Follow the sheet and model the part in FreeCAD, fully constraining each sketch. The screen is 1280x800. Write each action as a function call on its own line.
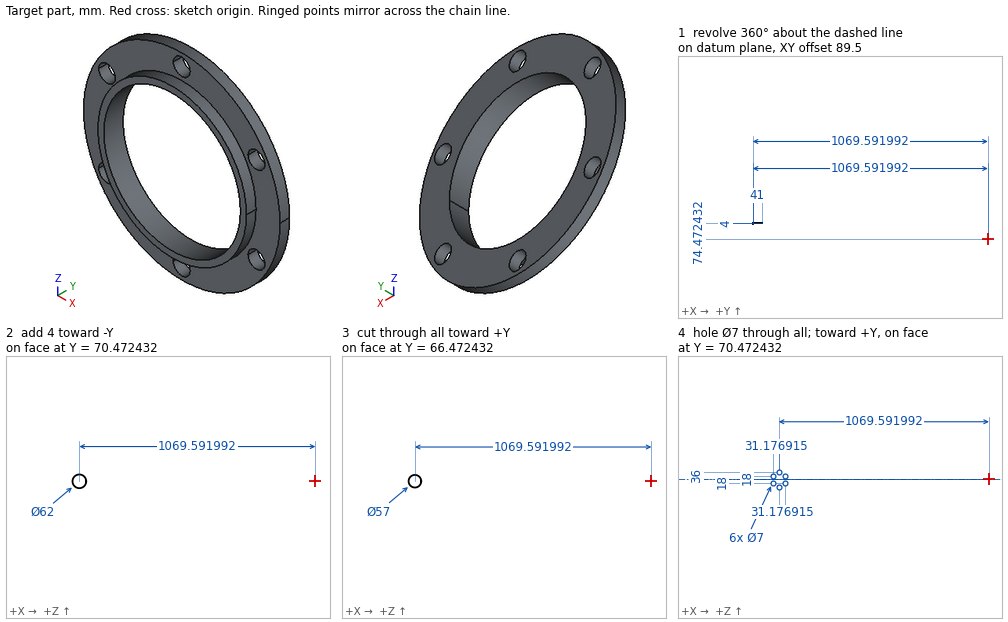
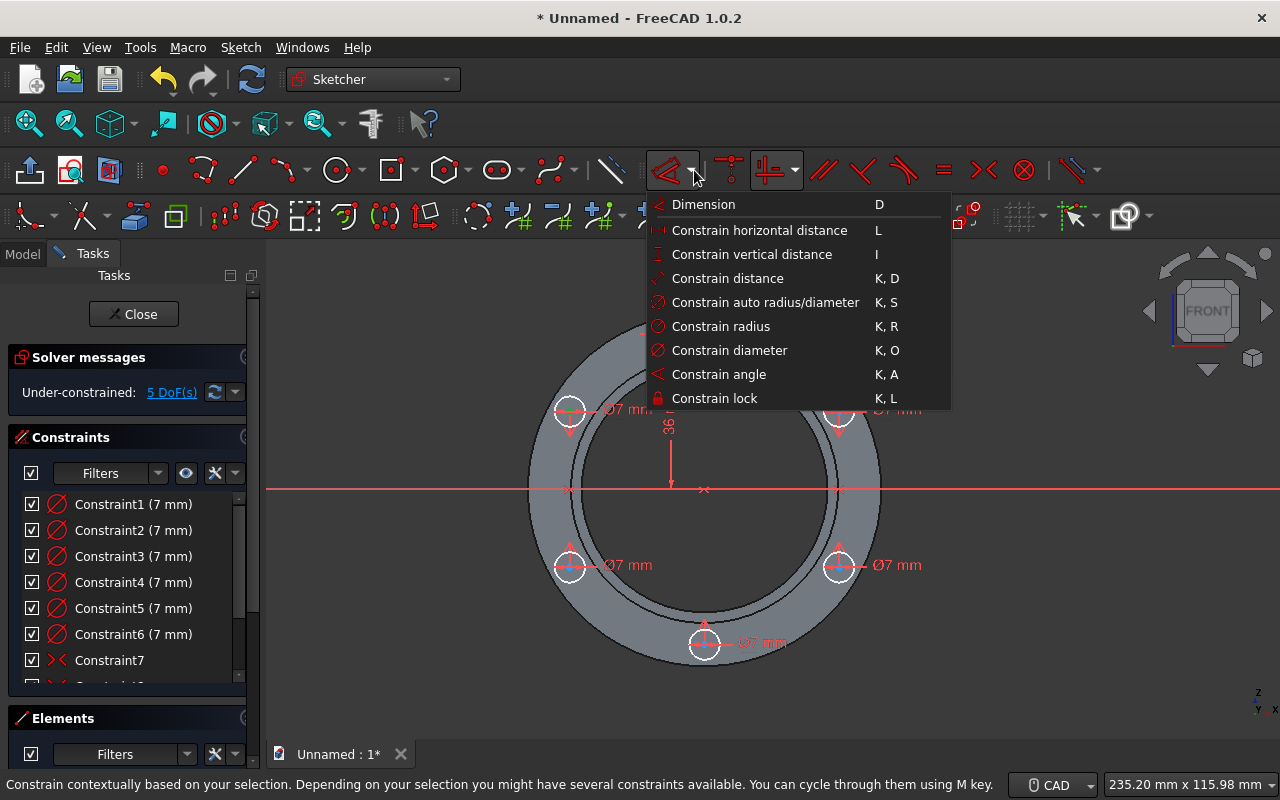
click(799, 254)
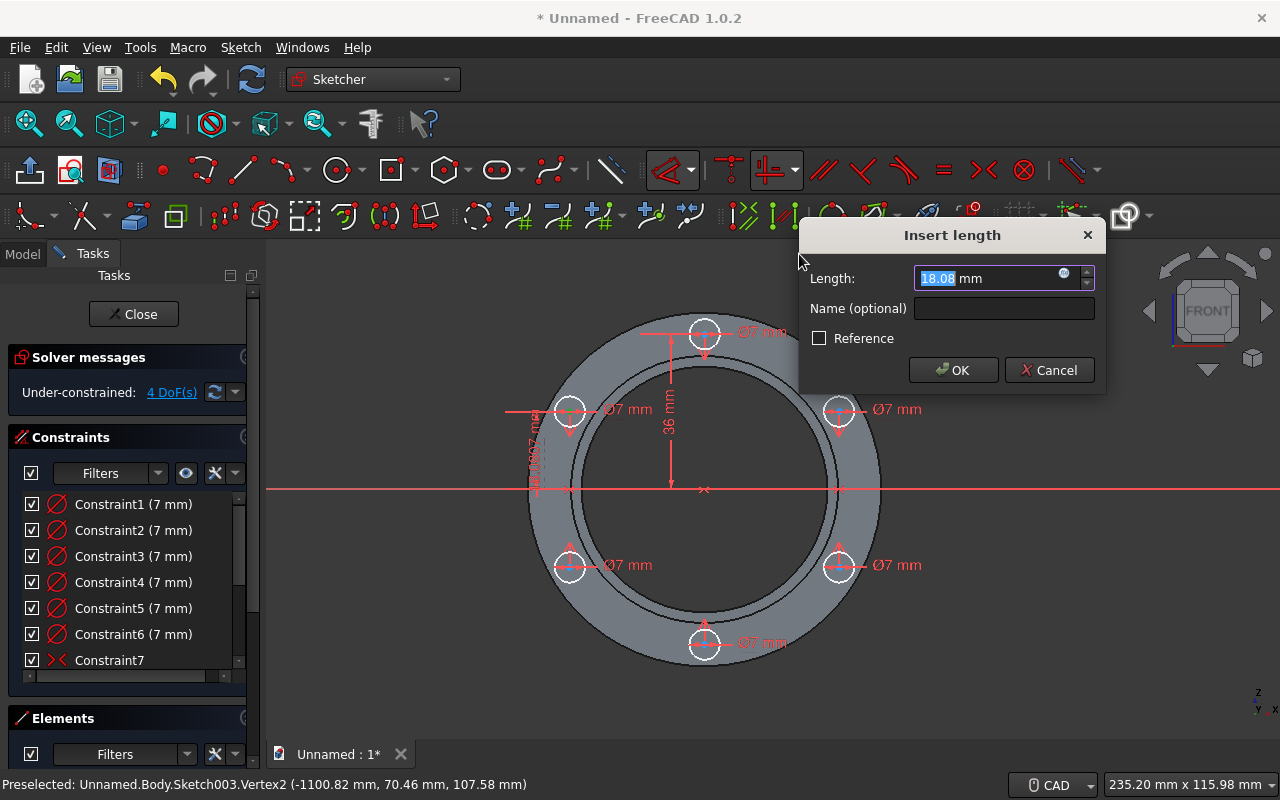
text(18)
key(Return)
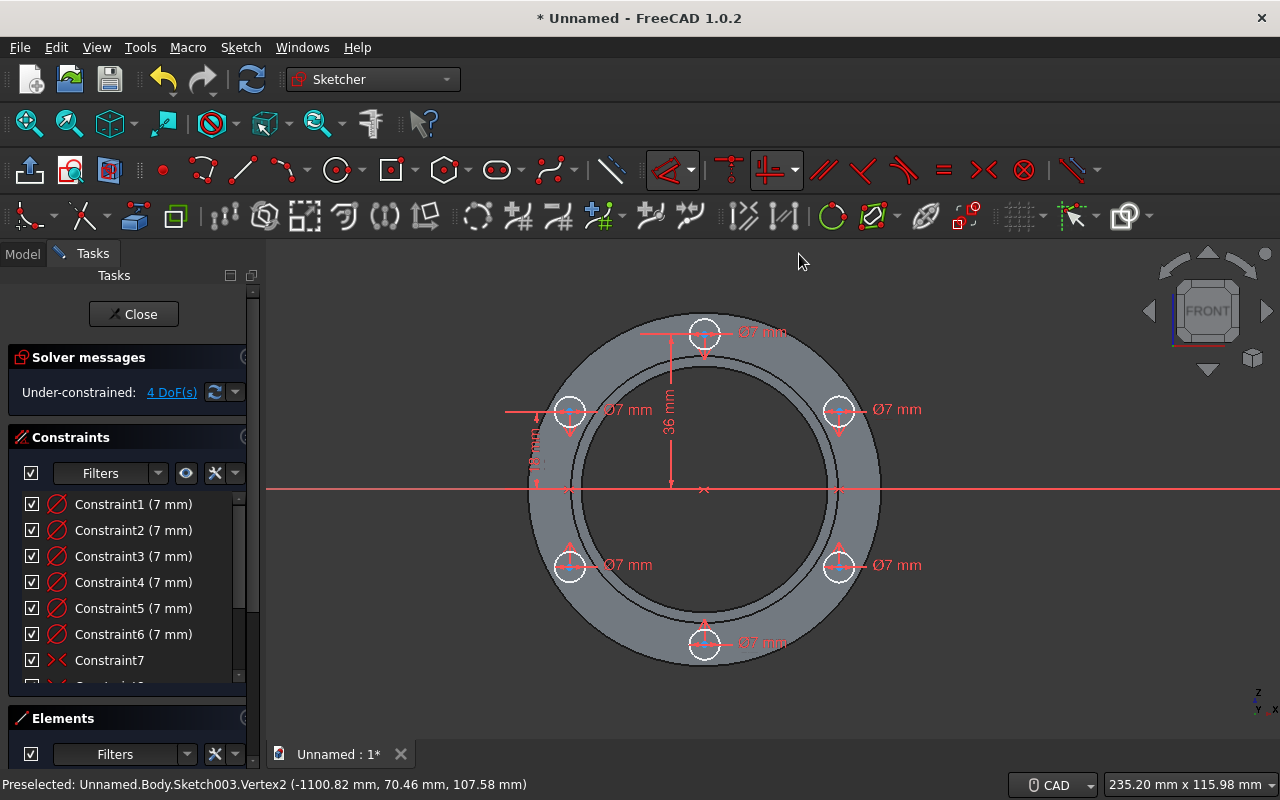
click(839, 567)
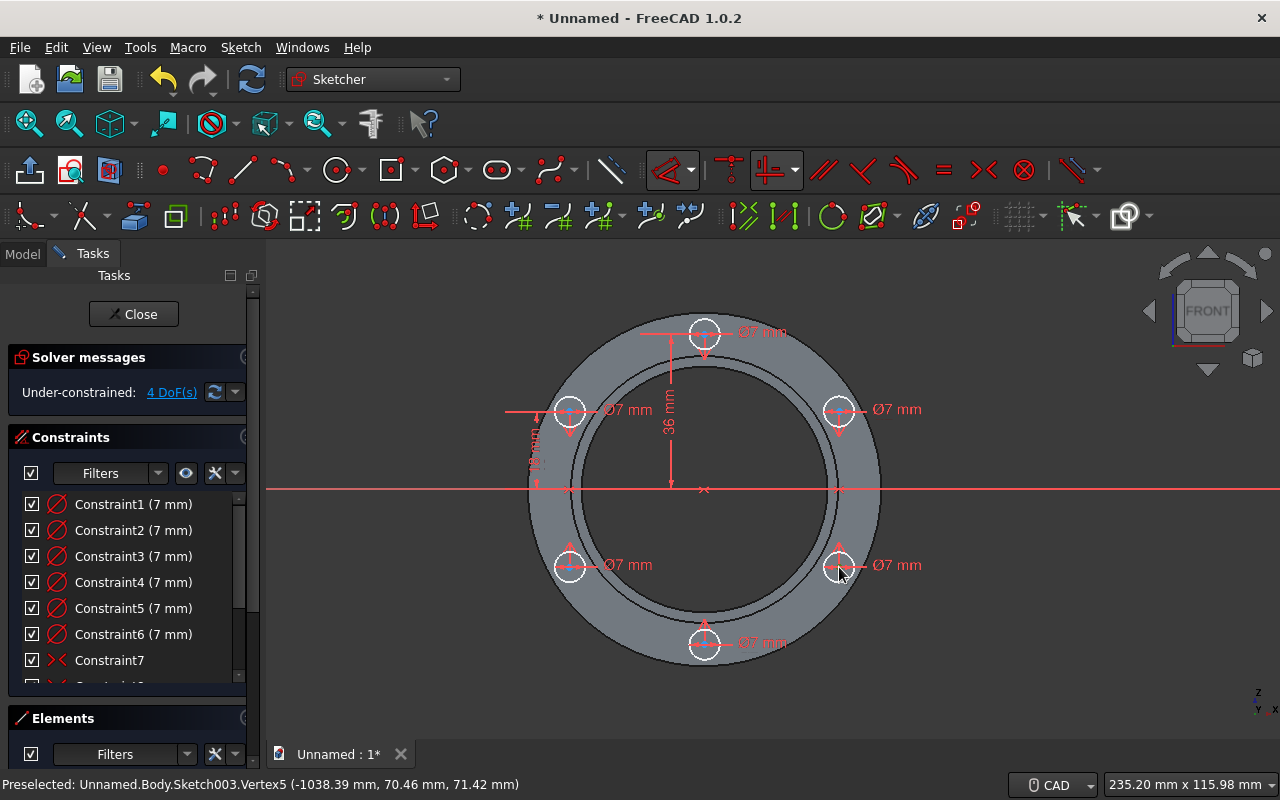
click(694, 170)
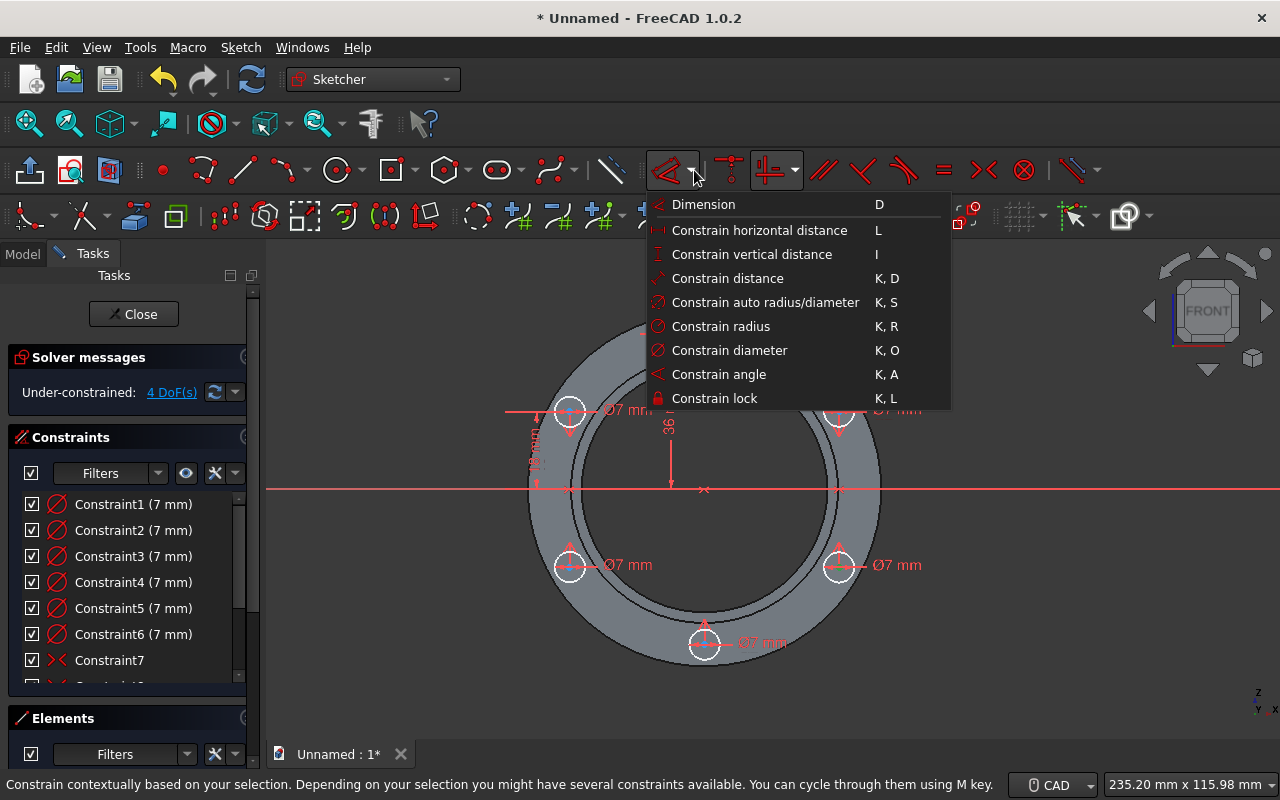
click(799, 254)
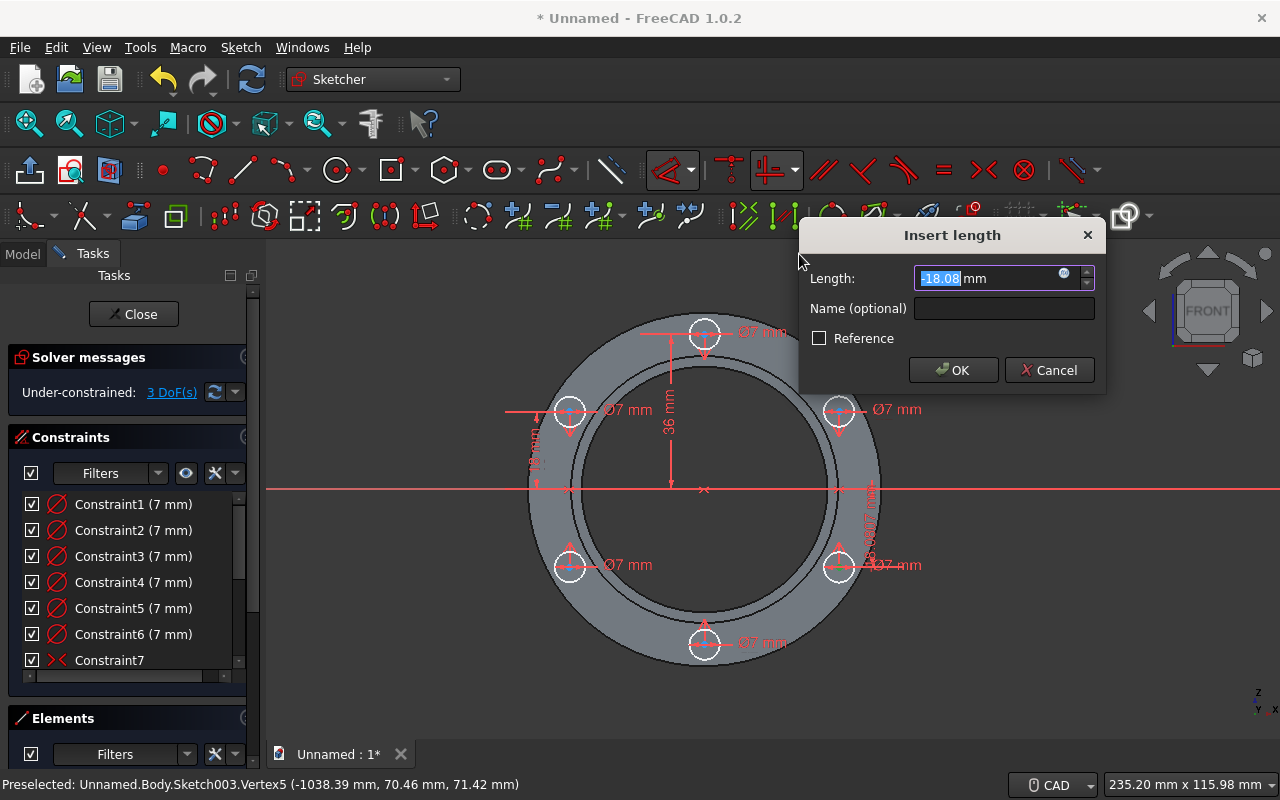
text(-18)
key(Return)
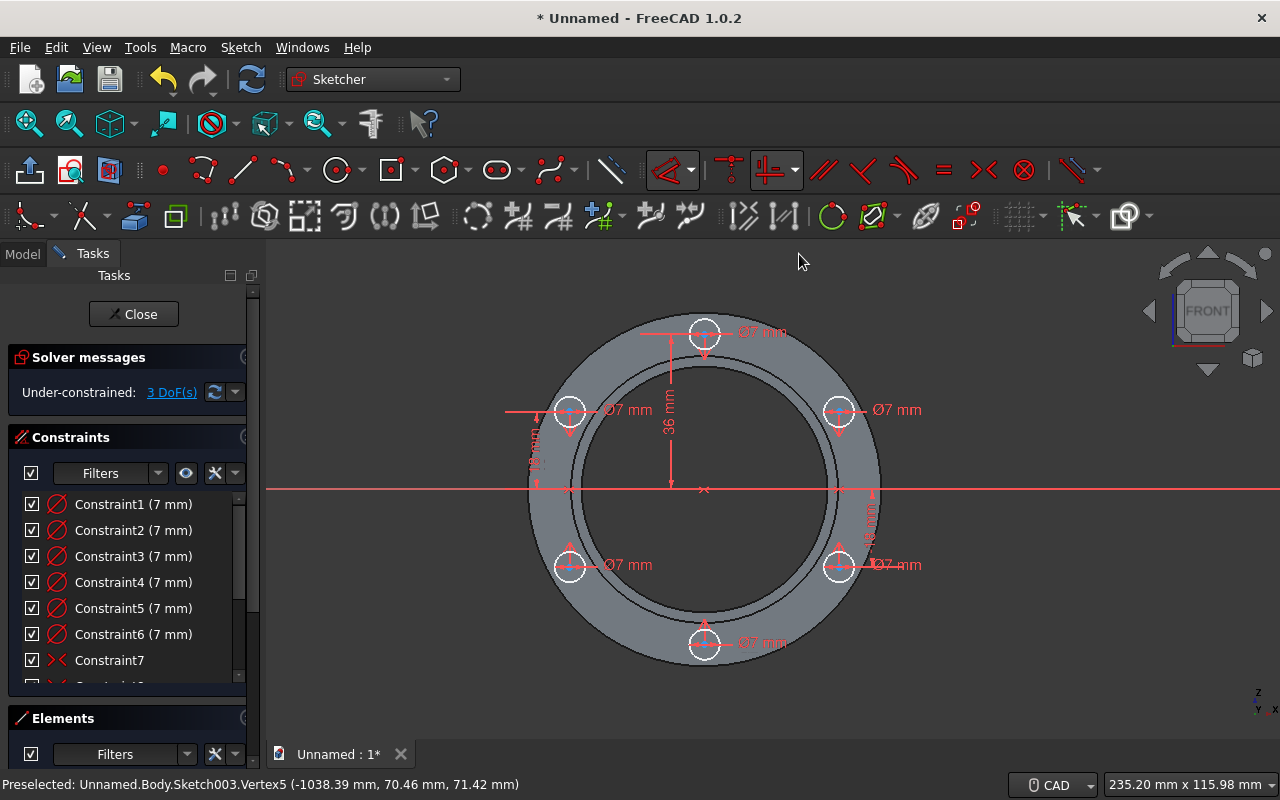
click(705, 334)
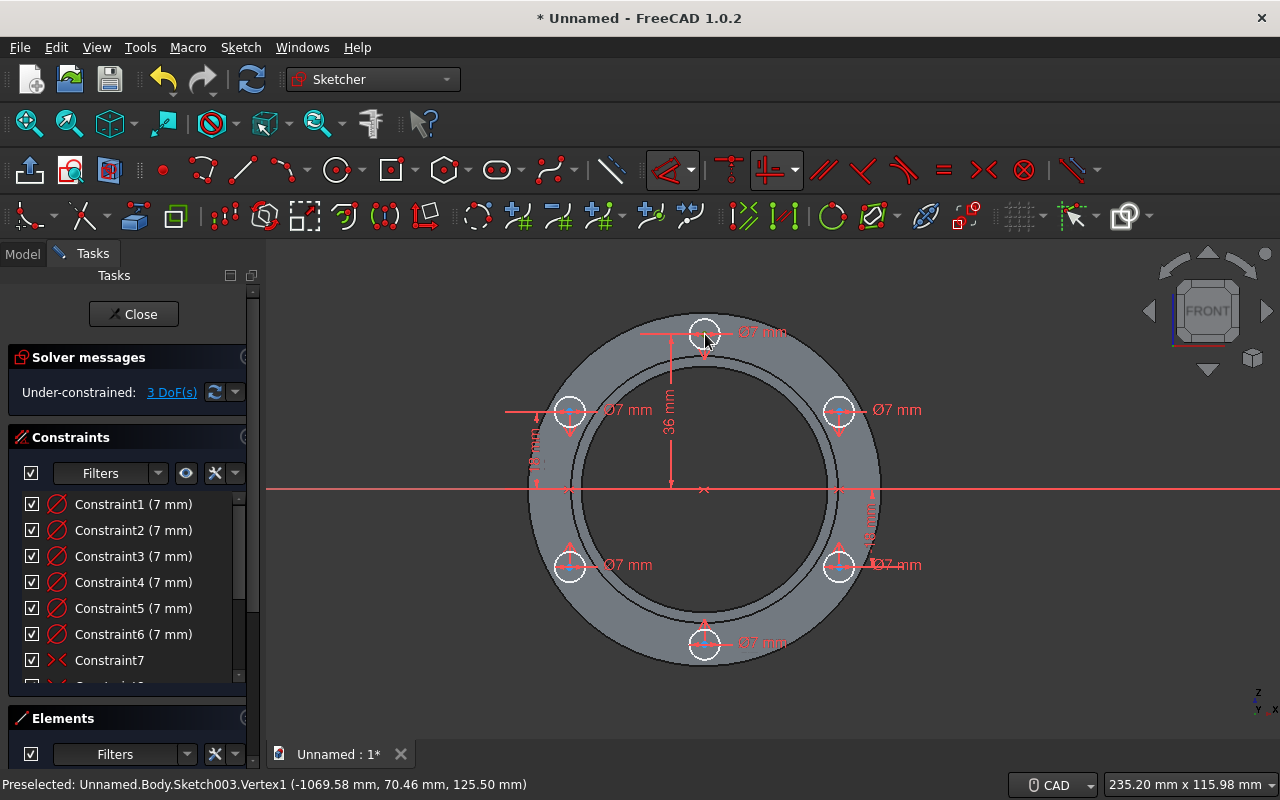
click(570, 412)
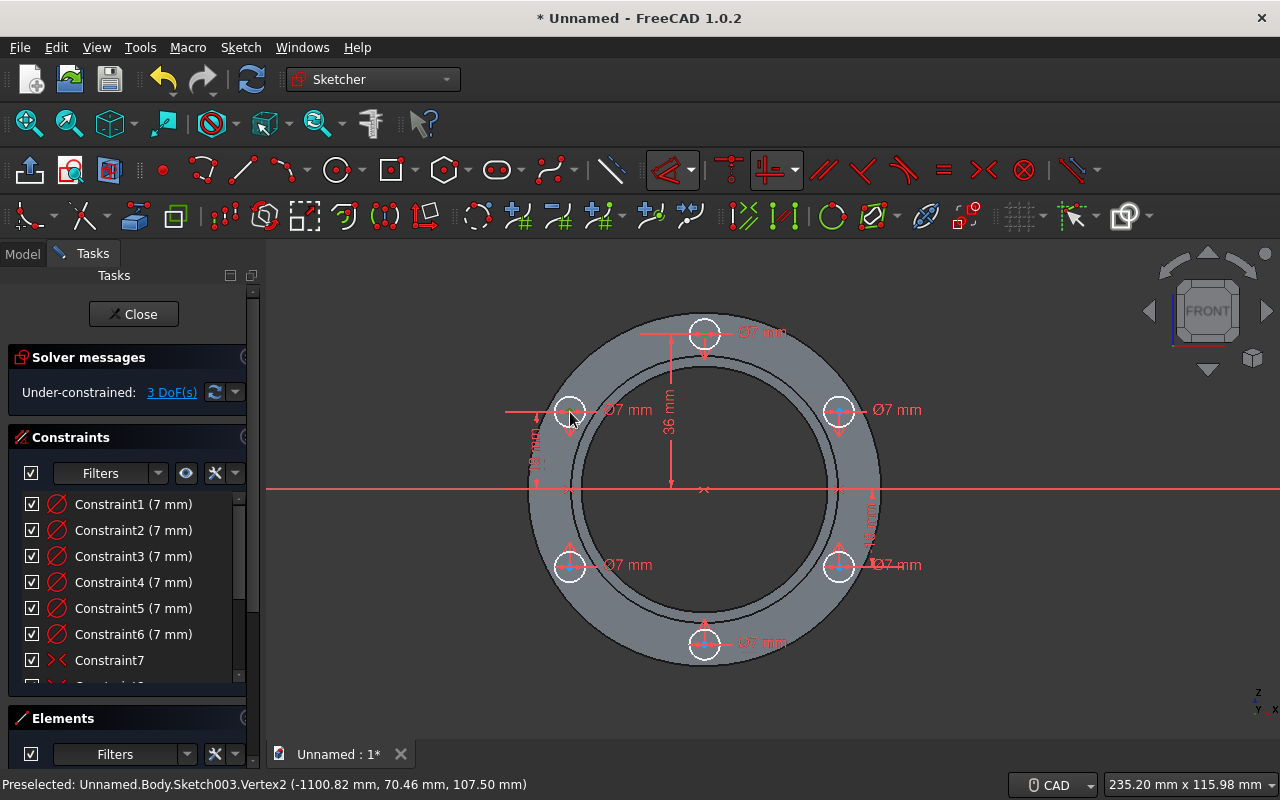
click(694, 170)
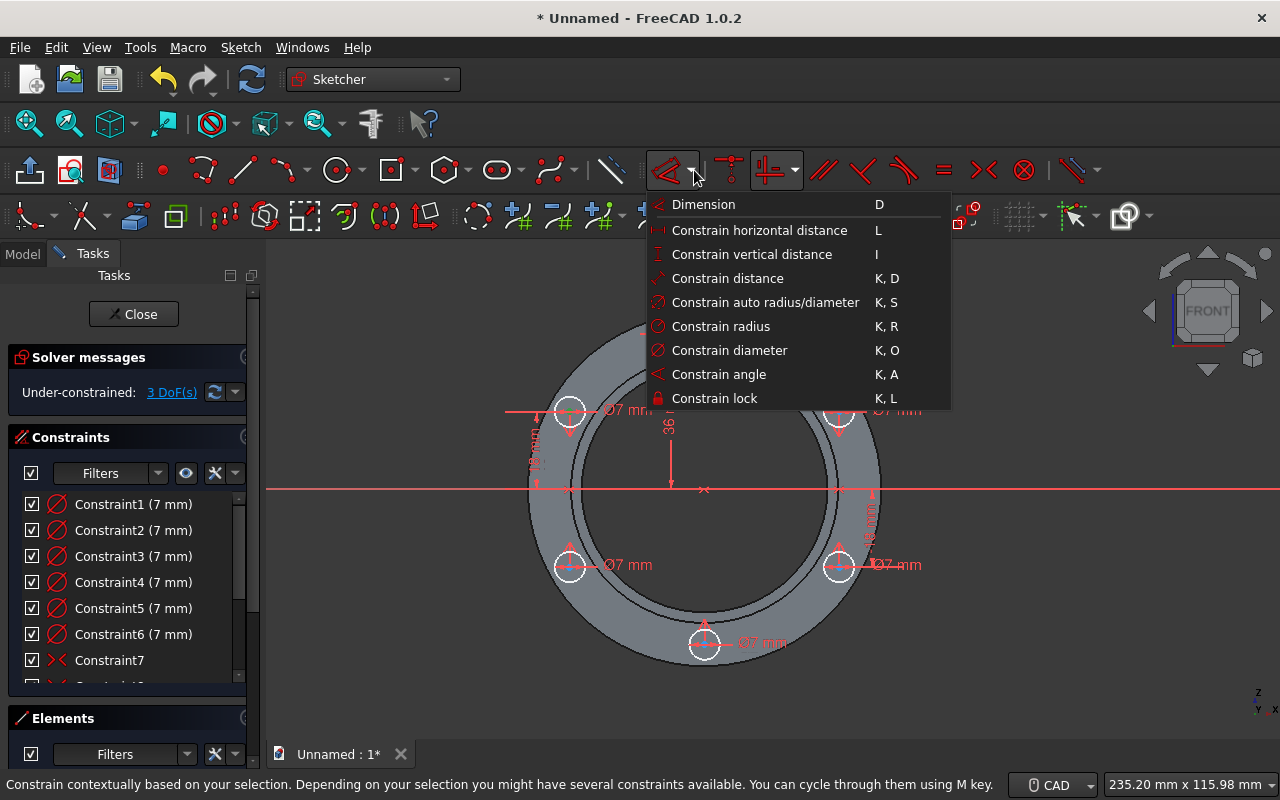
click(799, 230)